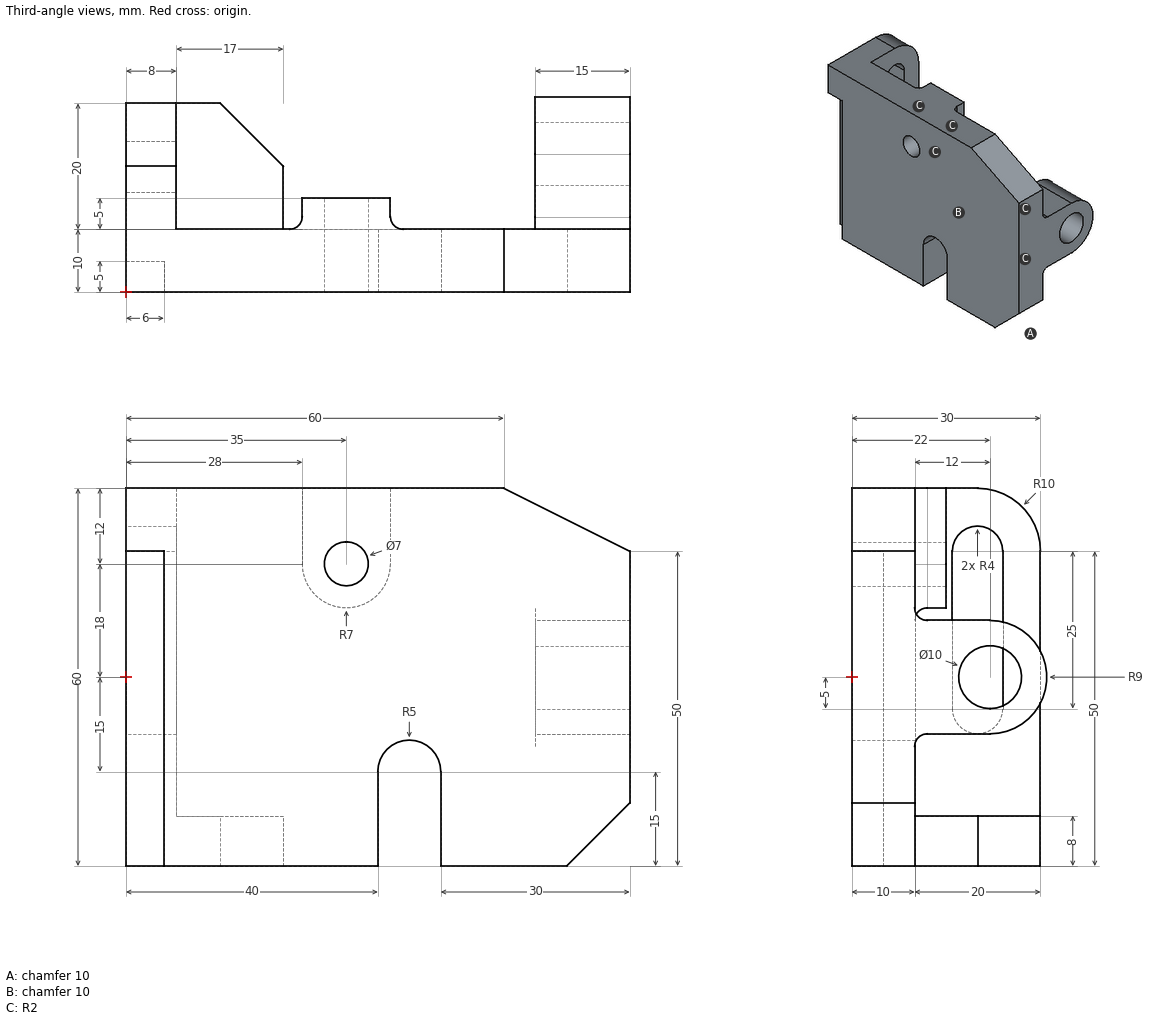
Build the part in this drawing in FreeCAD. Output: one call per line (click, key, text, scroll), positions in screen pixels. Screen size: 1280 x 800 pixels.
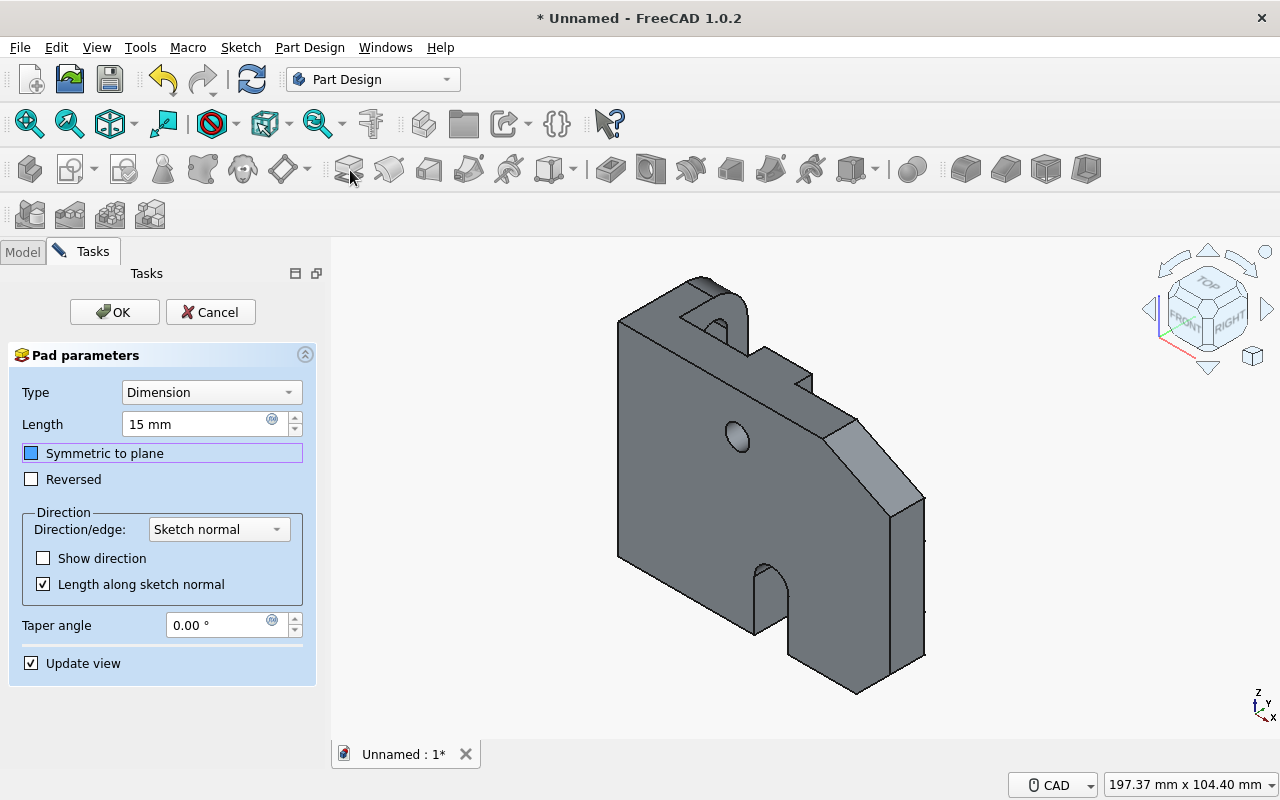
click(30, 479)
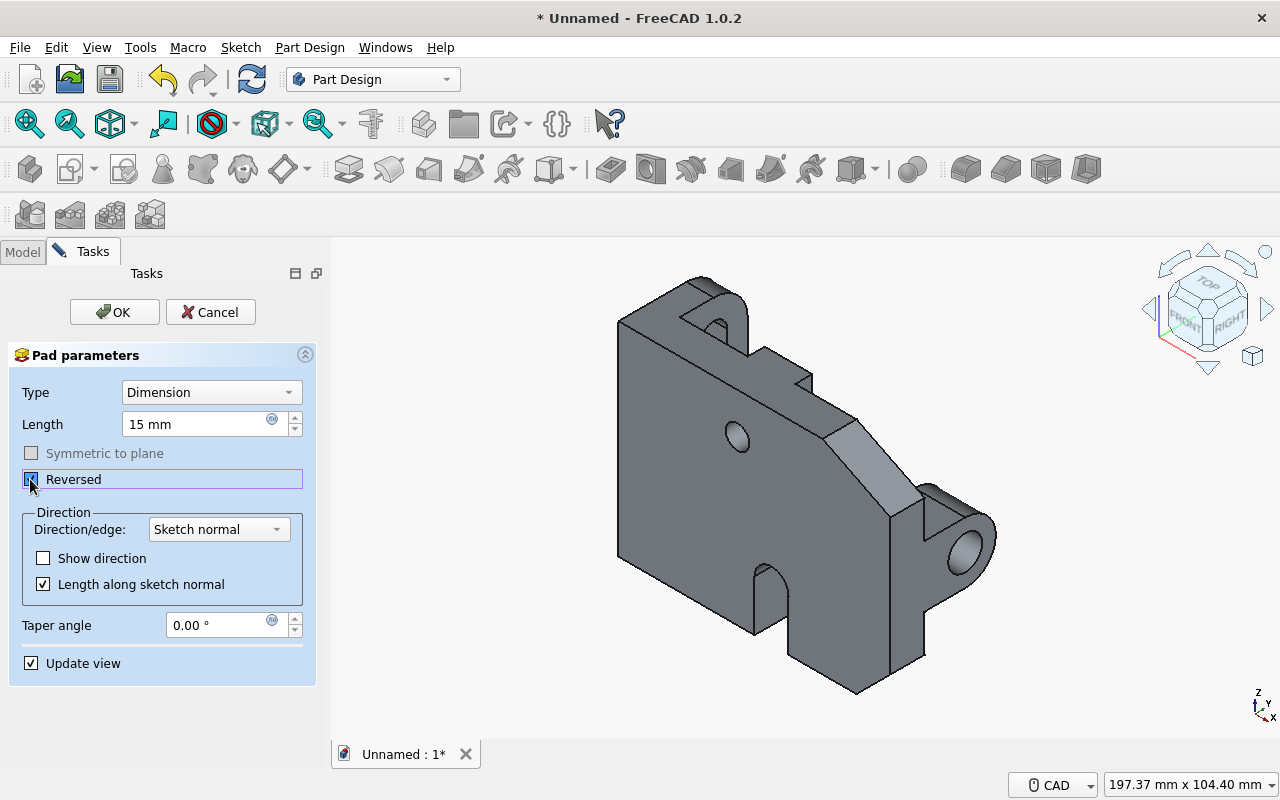
click(115, 312)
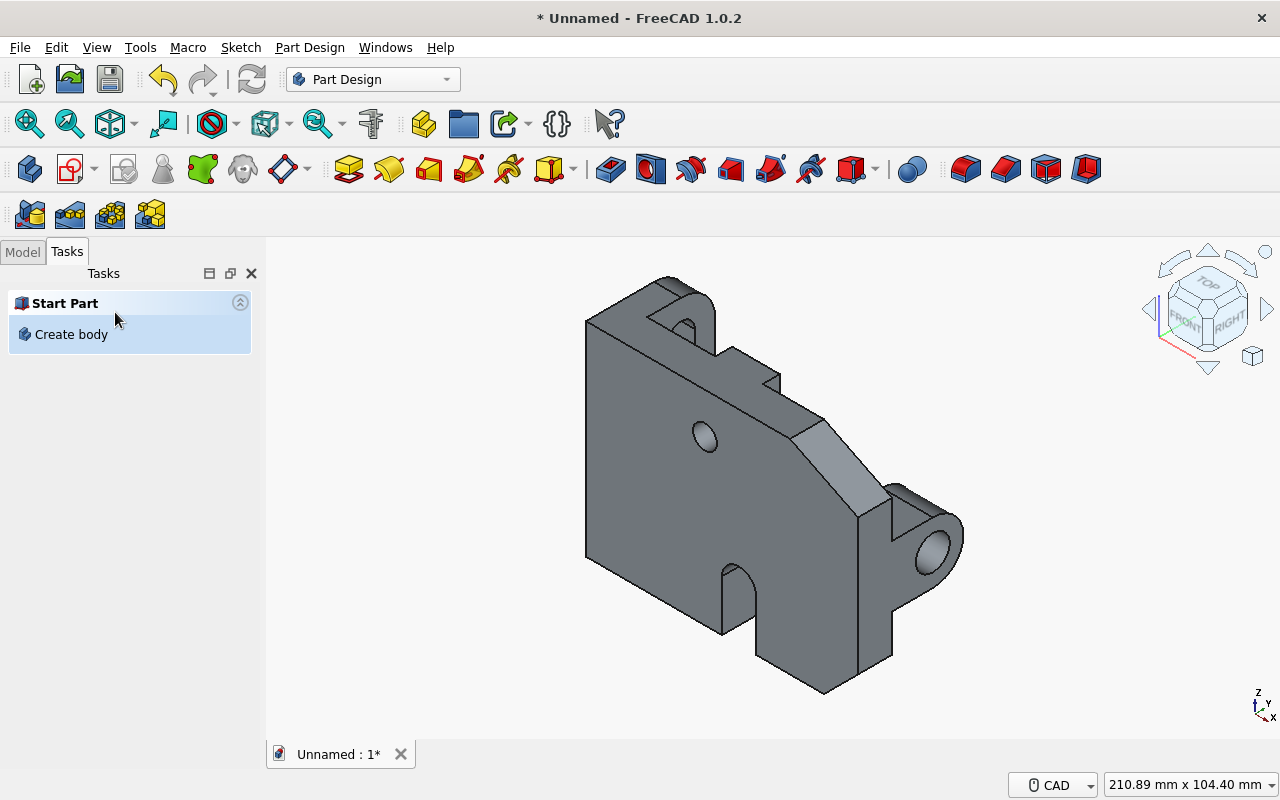
key(2)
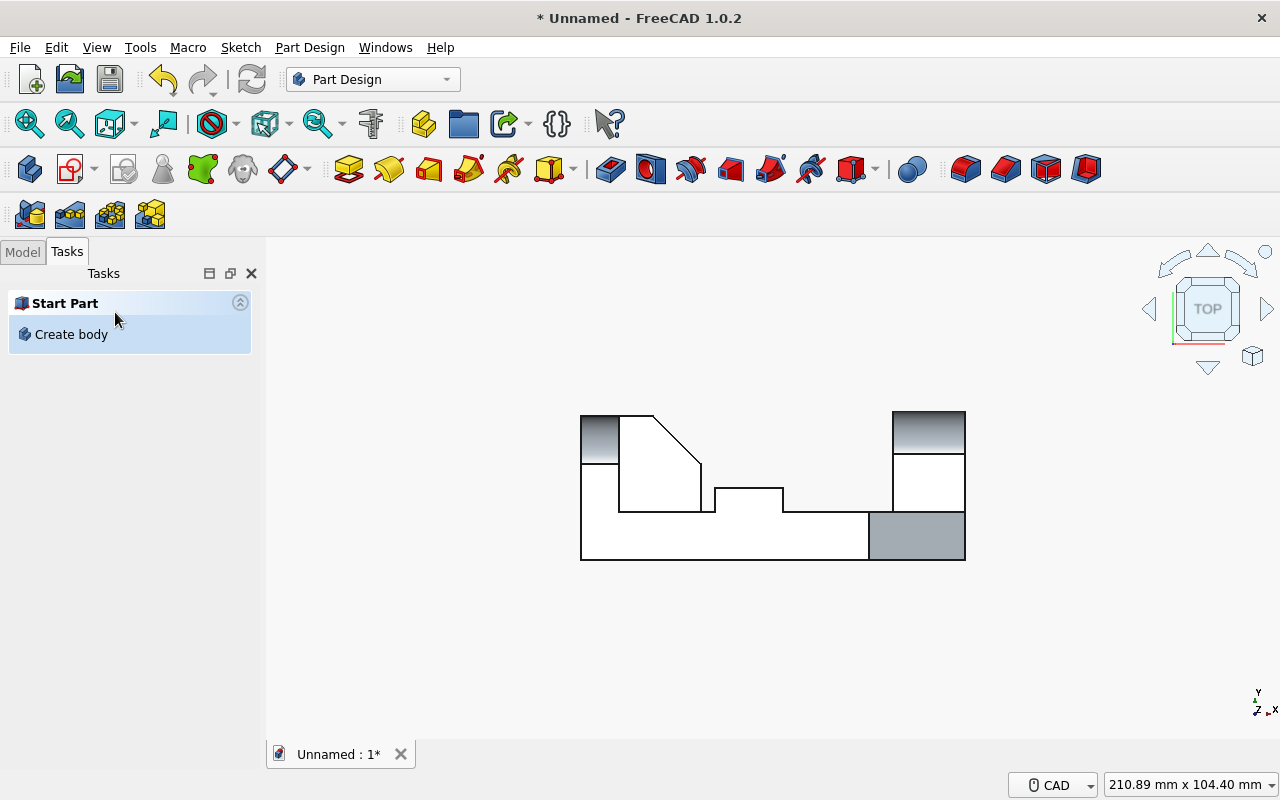
click(30, 124)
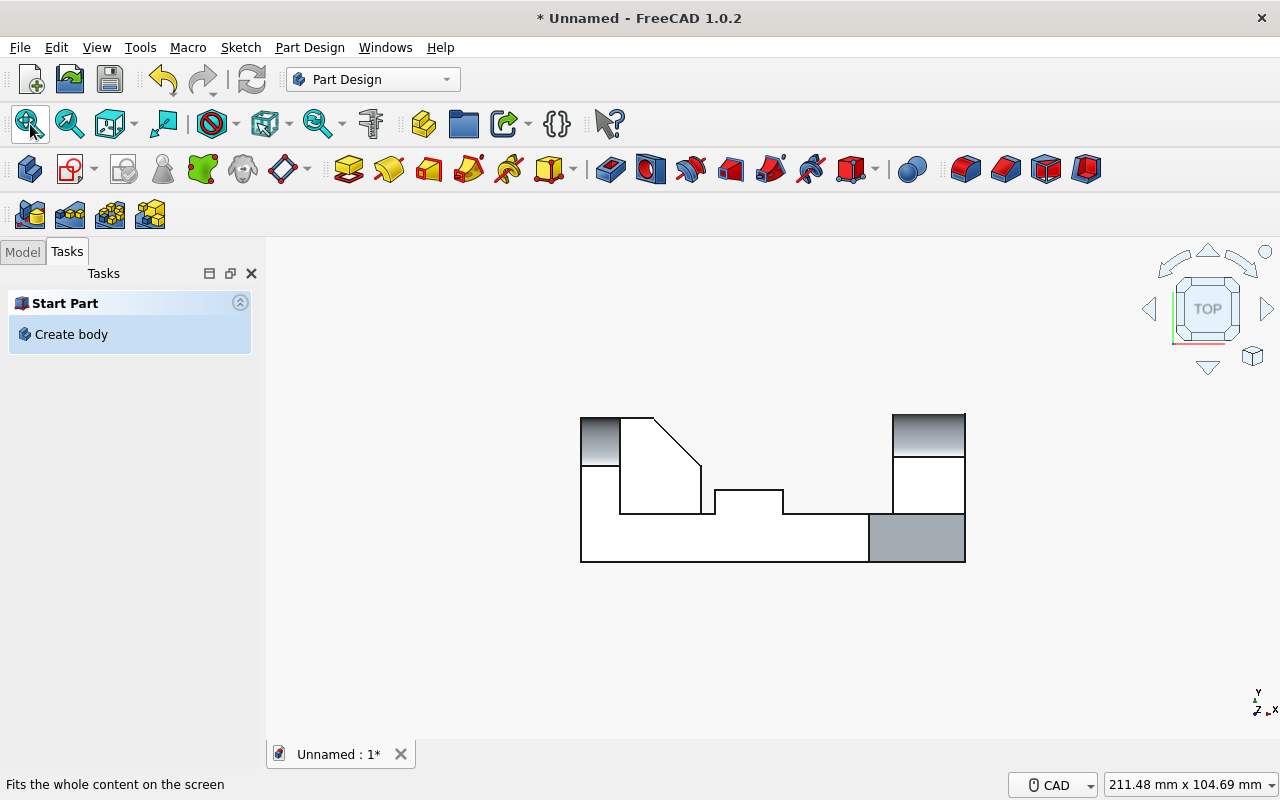
key(0)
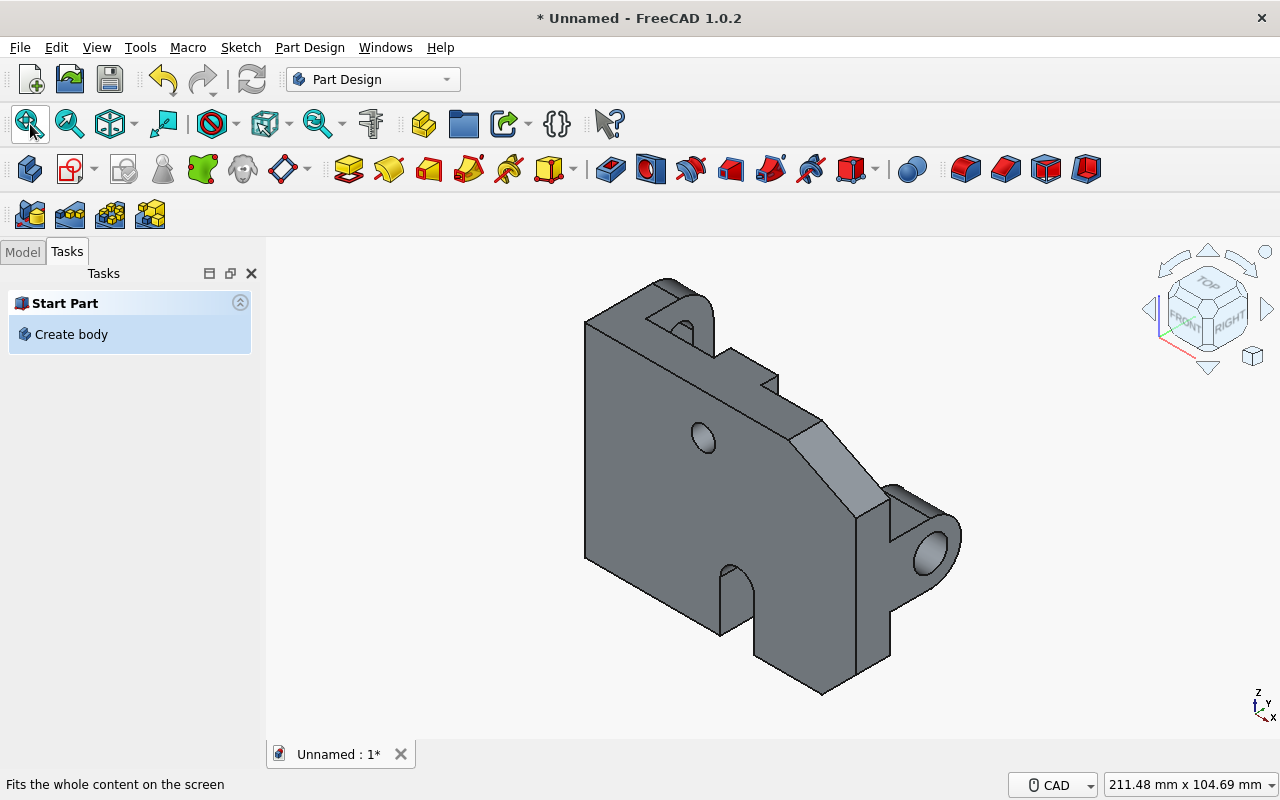
key(1)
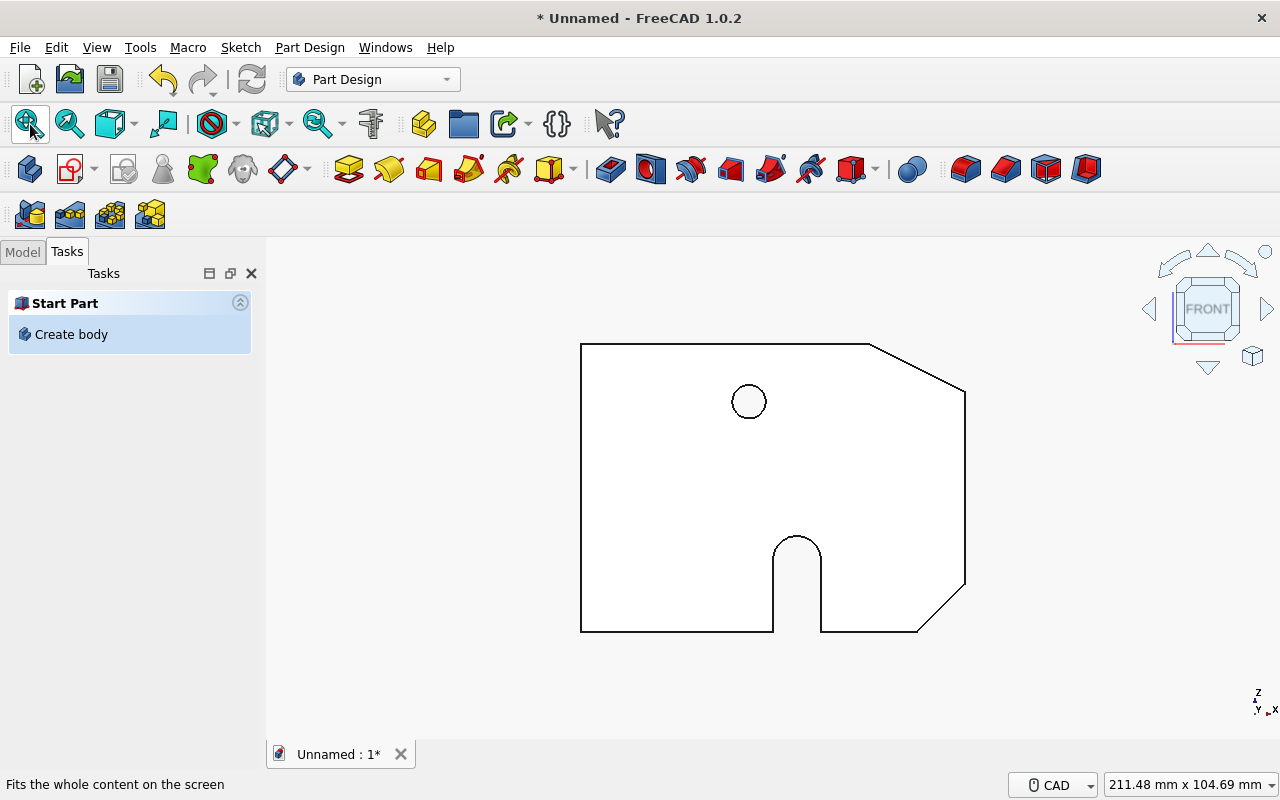
key(3)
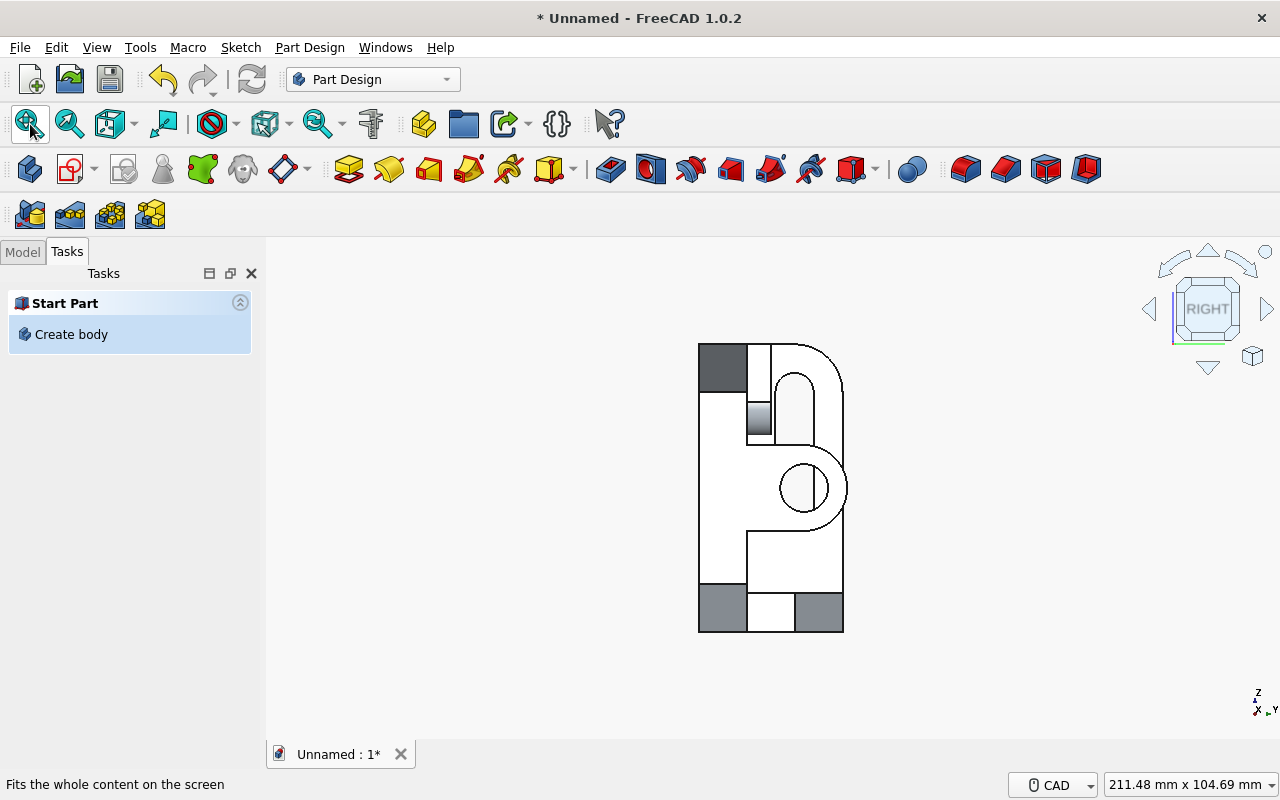
key(5)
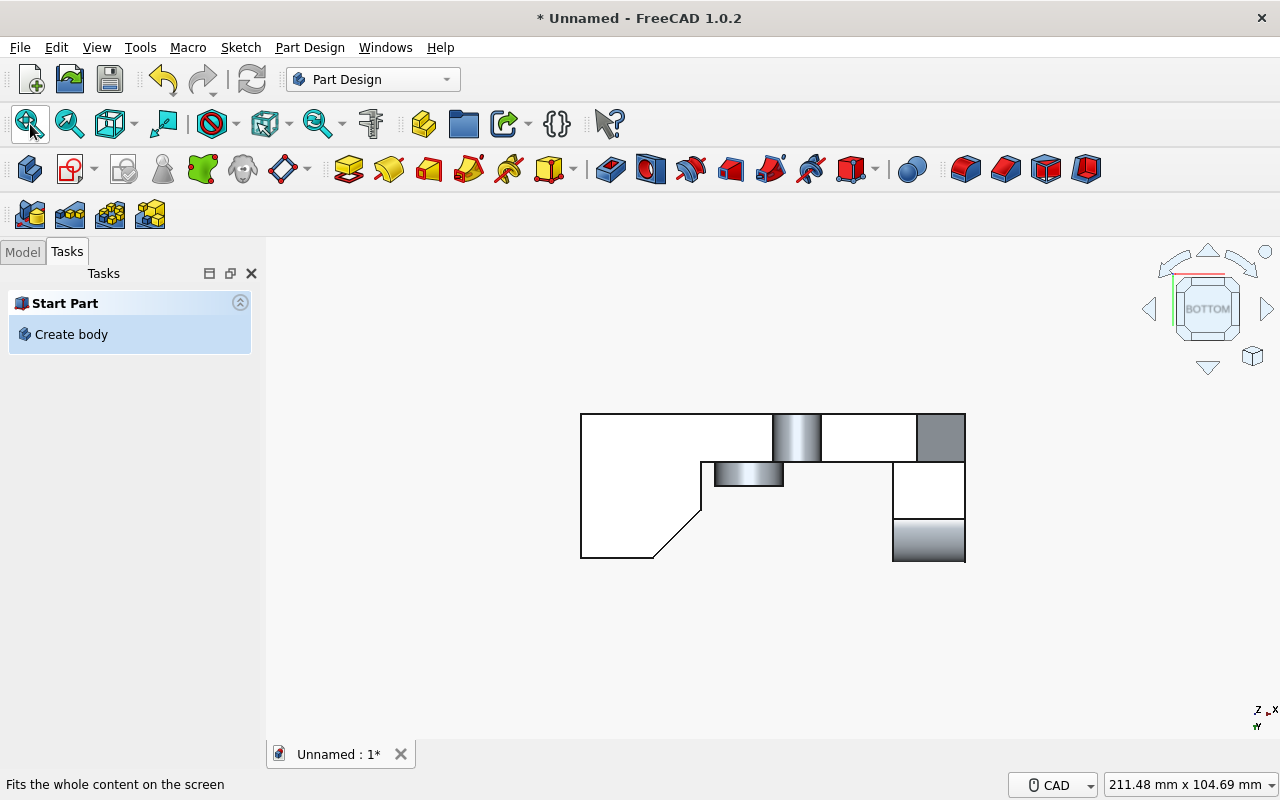
click(30, 124)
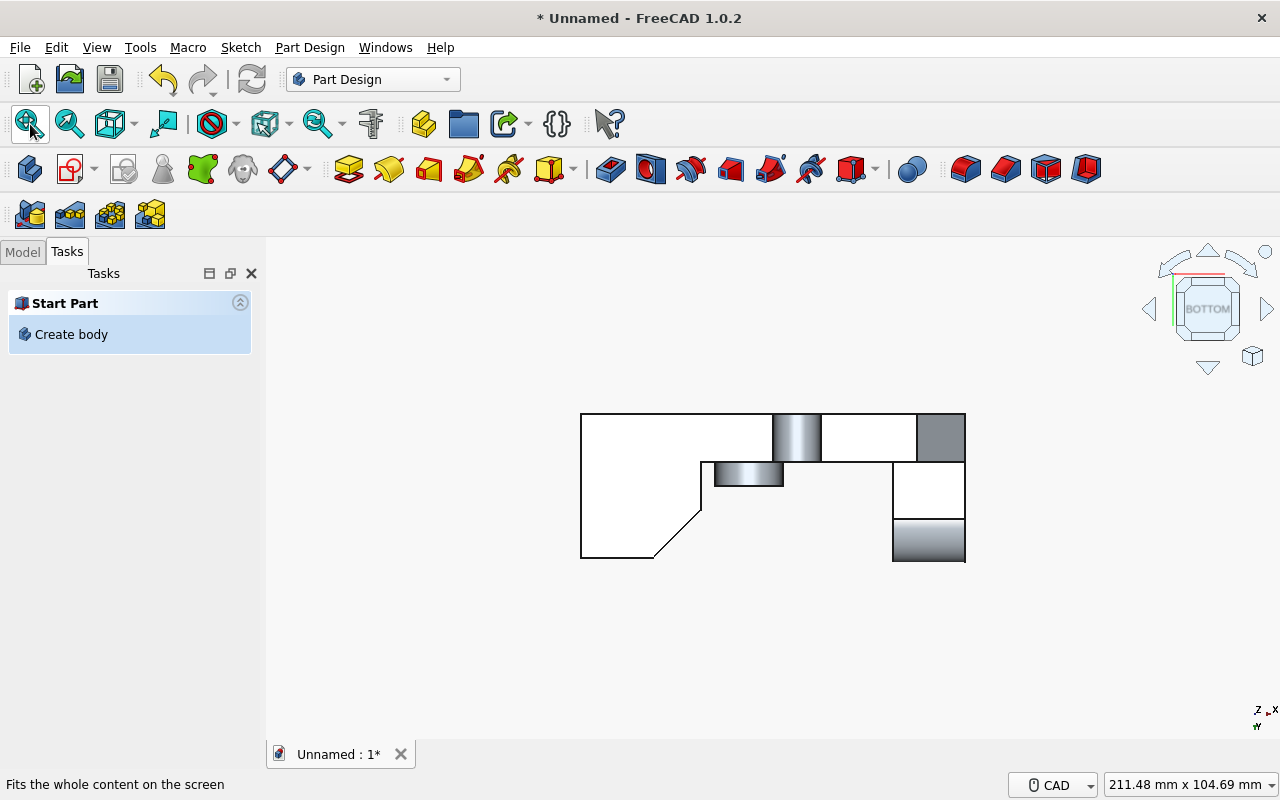
key(4)